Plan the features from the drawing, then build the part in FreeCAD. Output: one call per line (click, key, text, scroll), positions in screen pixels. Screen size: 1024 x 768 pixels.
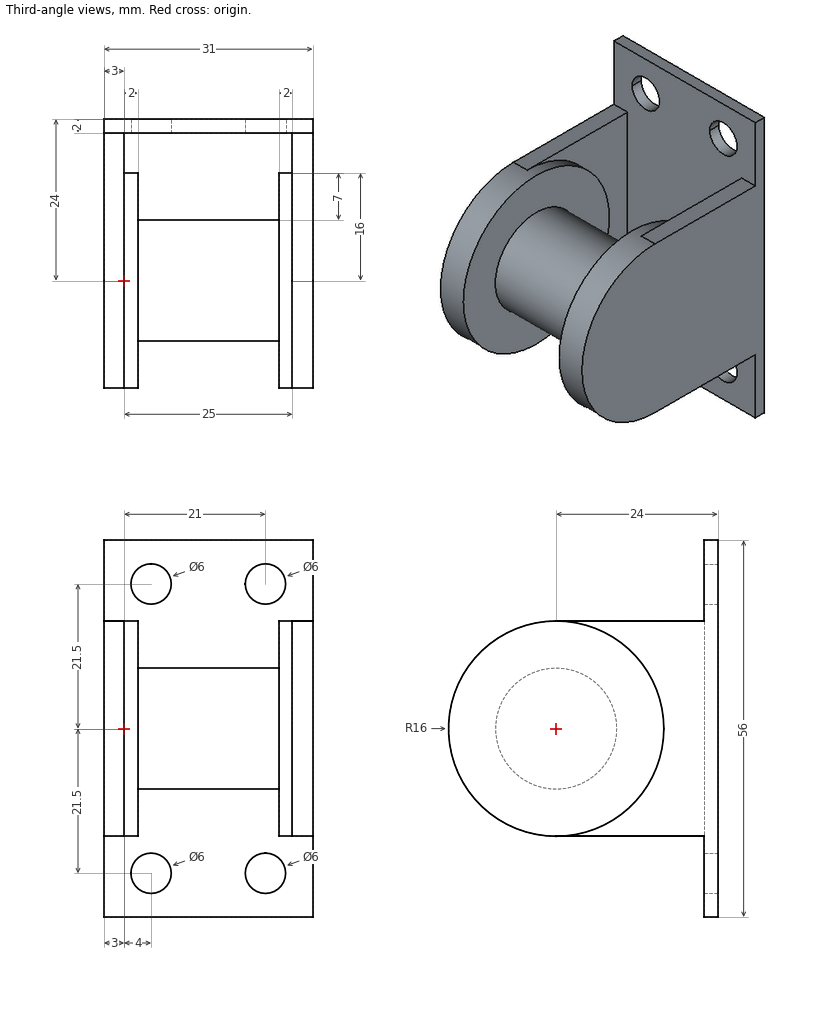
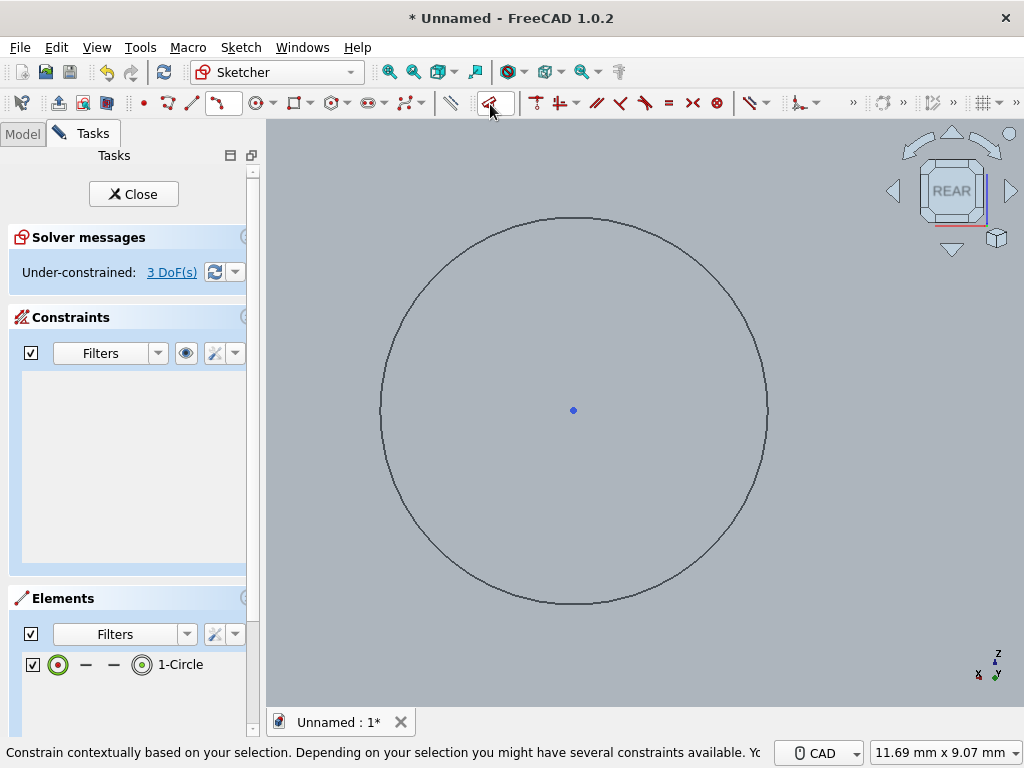
click(711, 274)
click(734, 251)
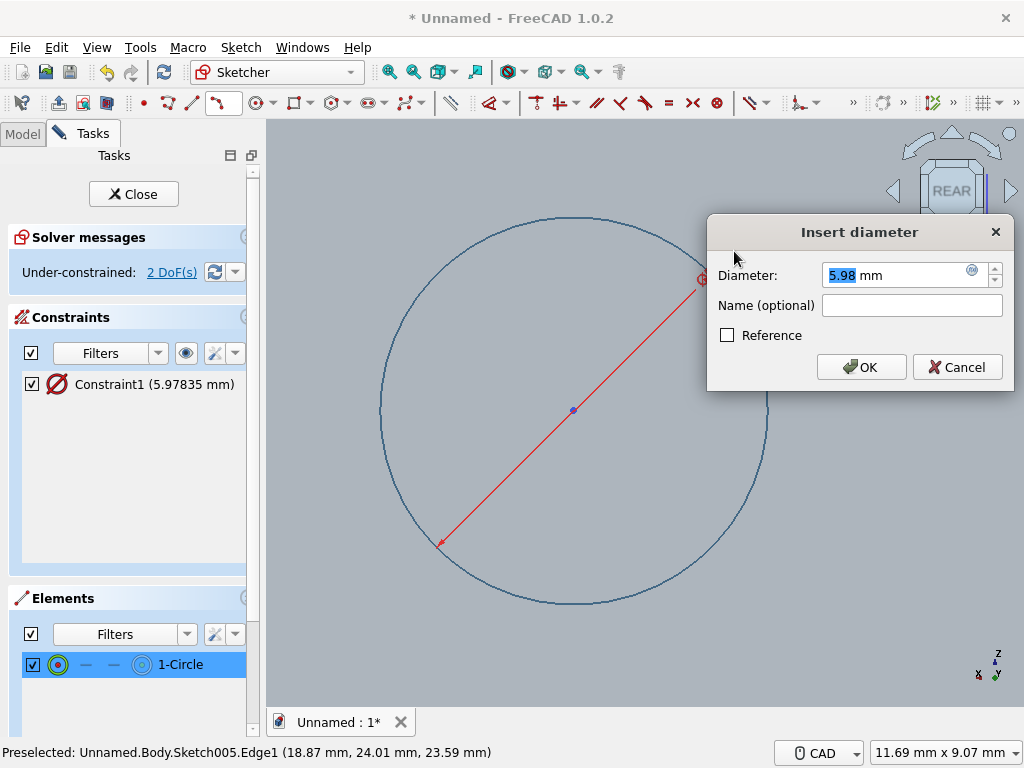
text(6)
key(Return)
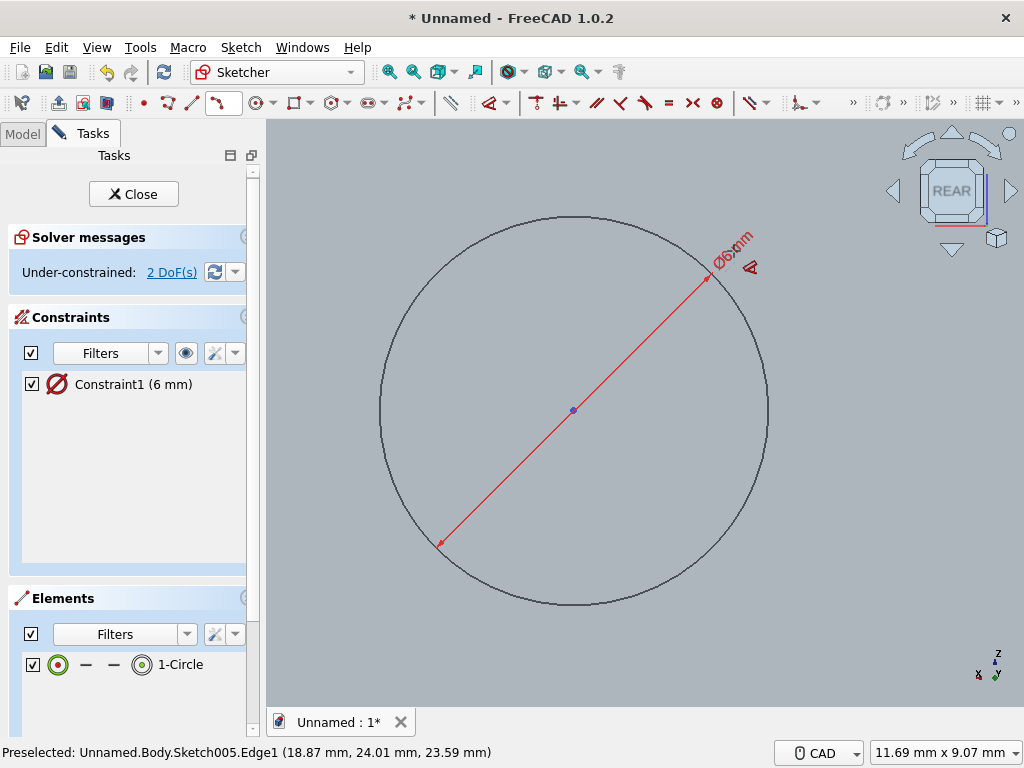
click(574, 411)
click(717, 377)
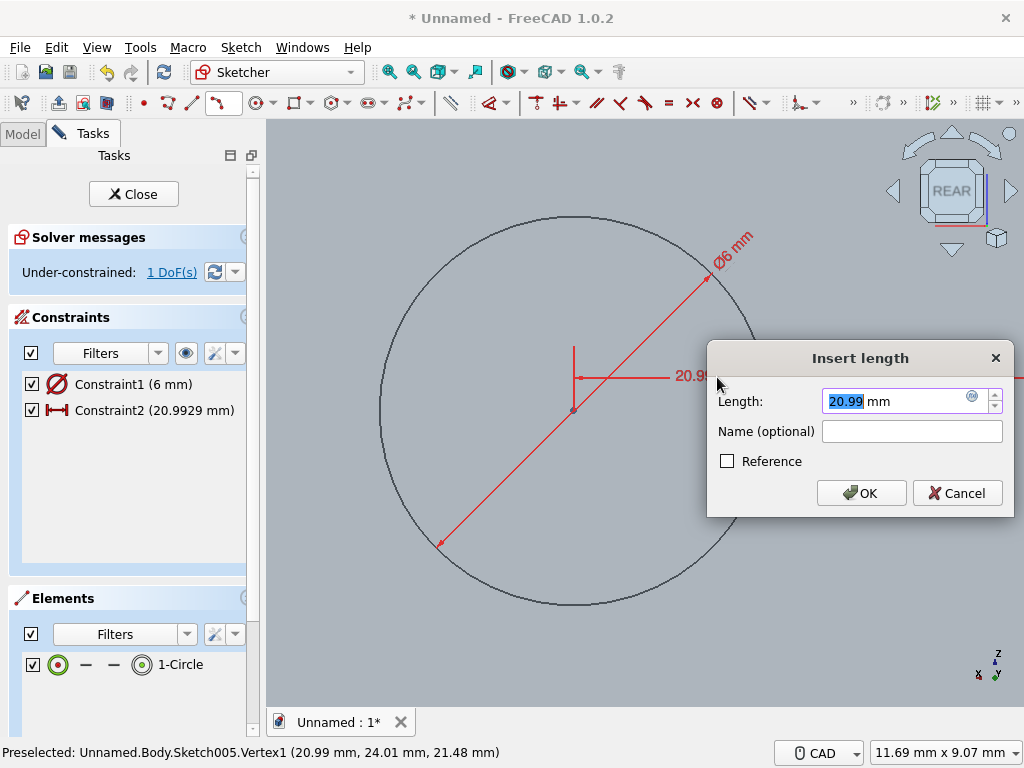
text(21)
key(Return)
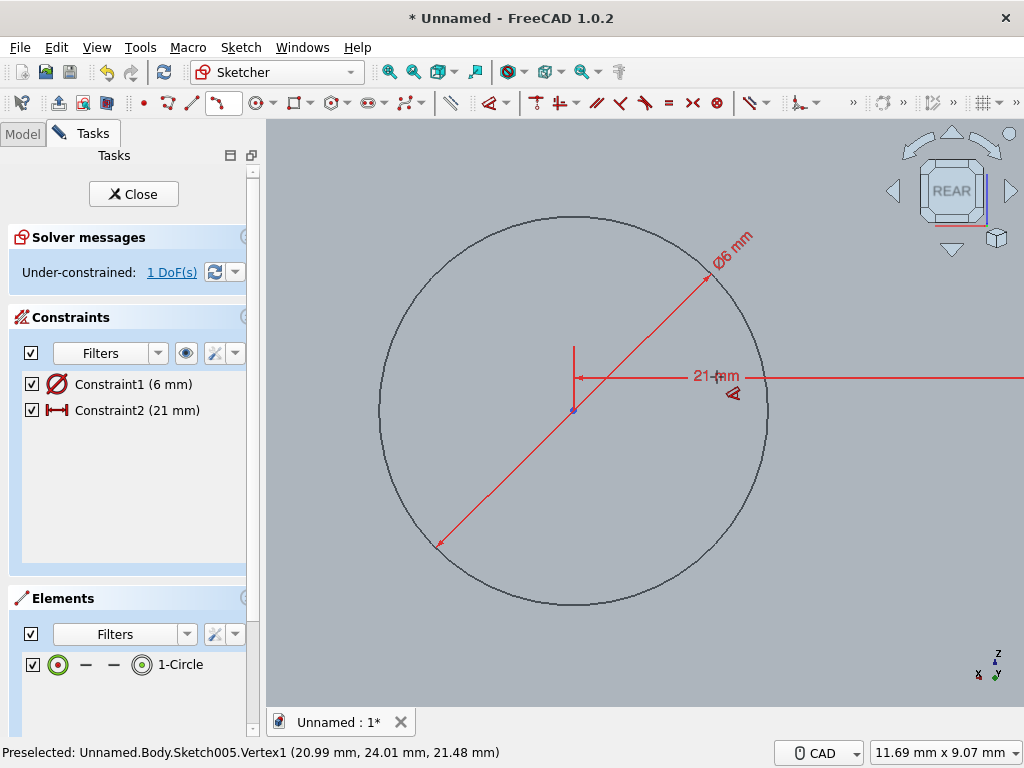
click(574, 411)
click(540, 545)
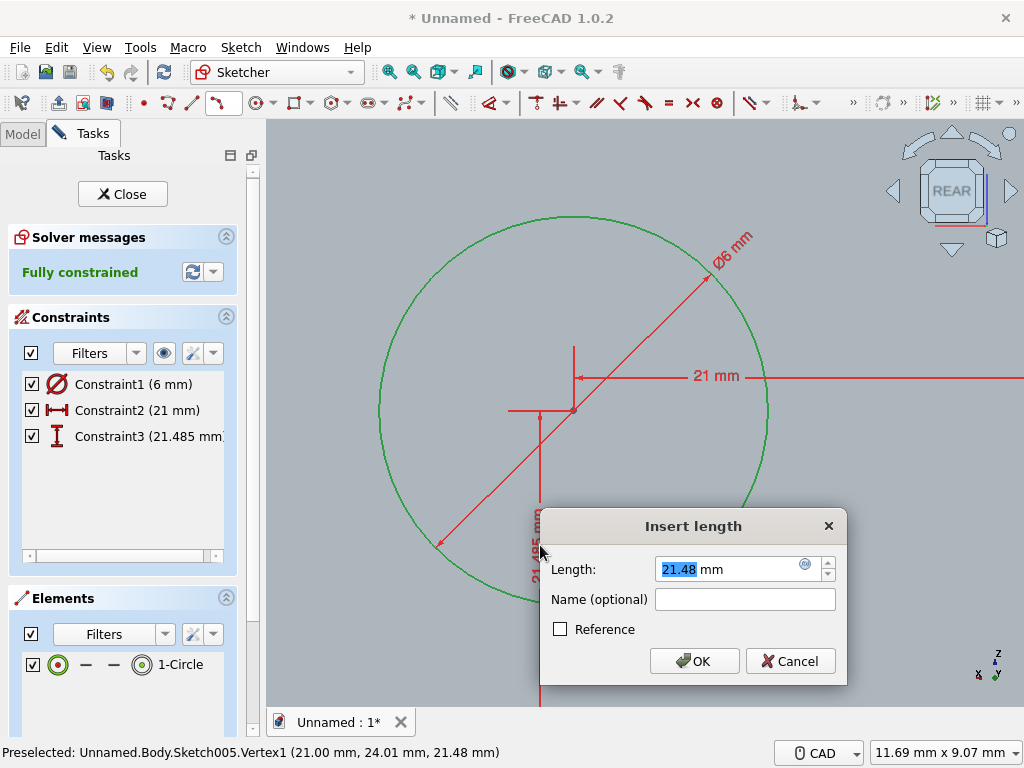
text(21.5)
key(Return)
key(Escape)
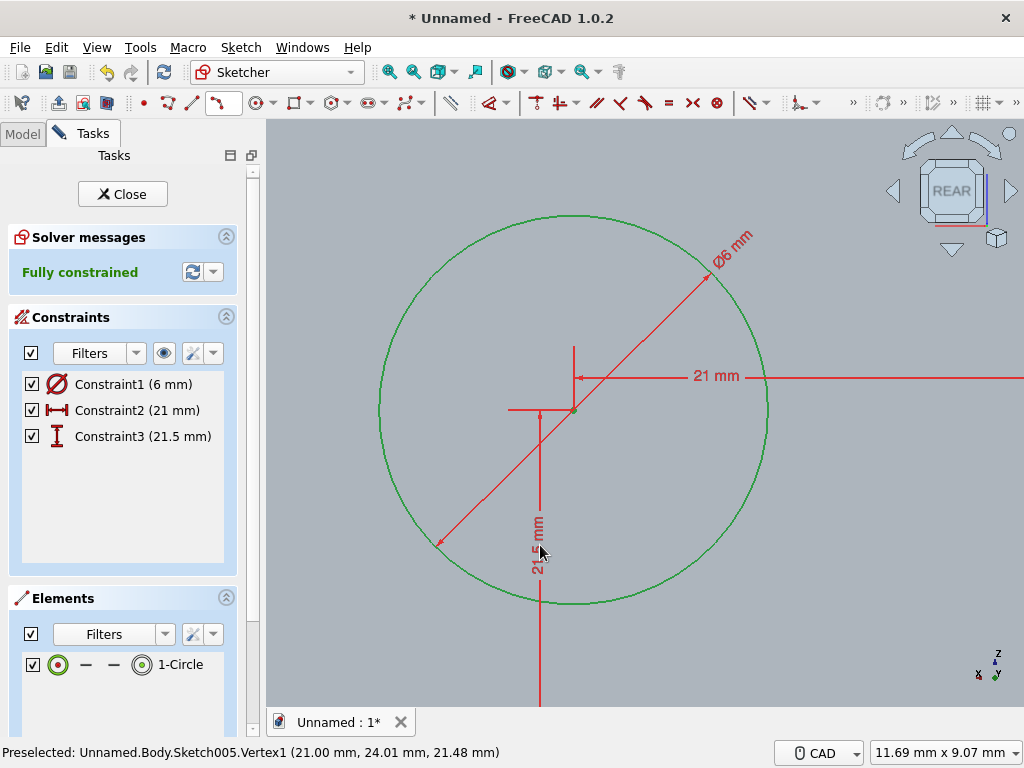
click(123, 194)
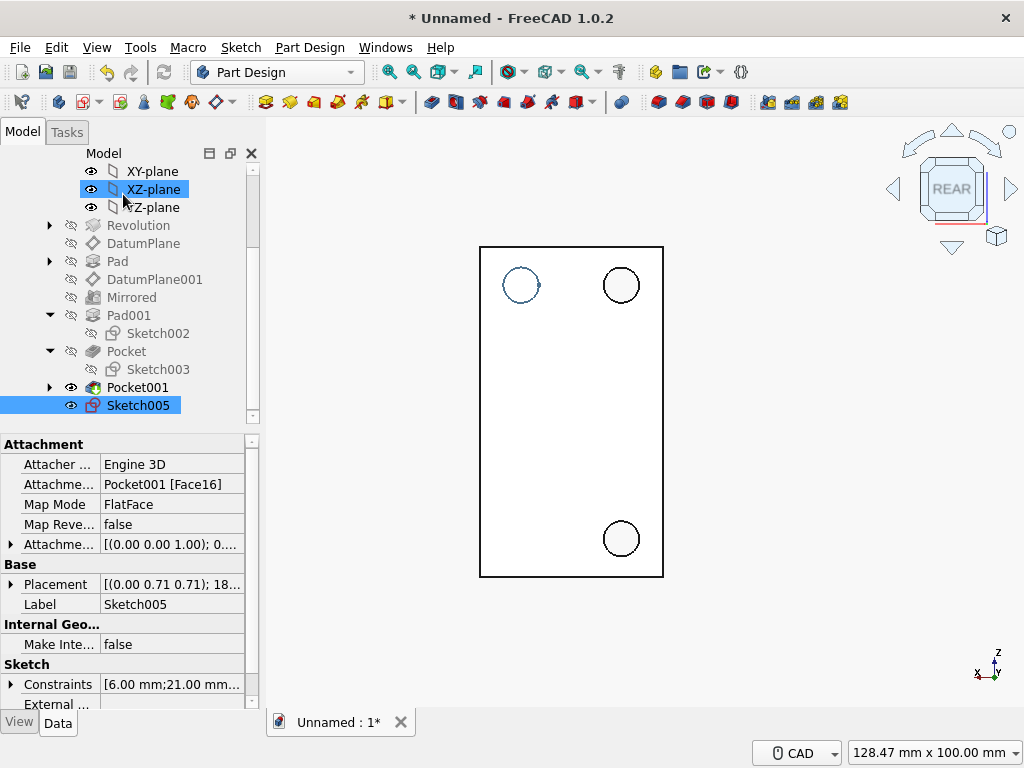
click(432, 102)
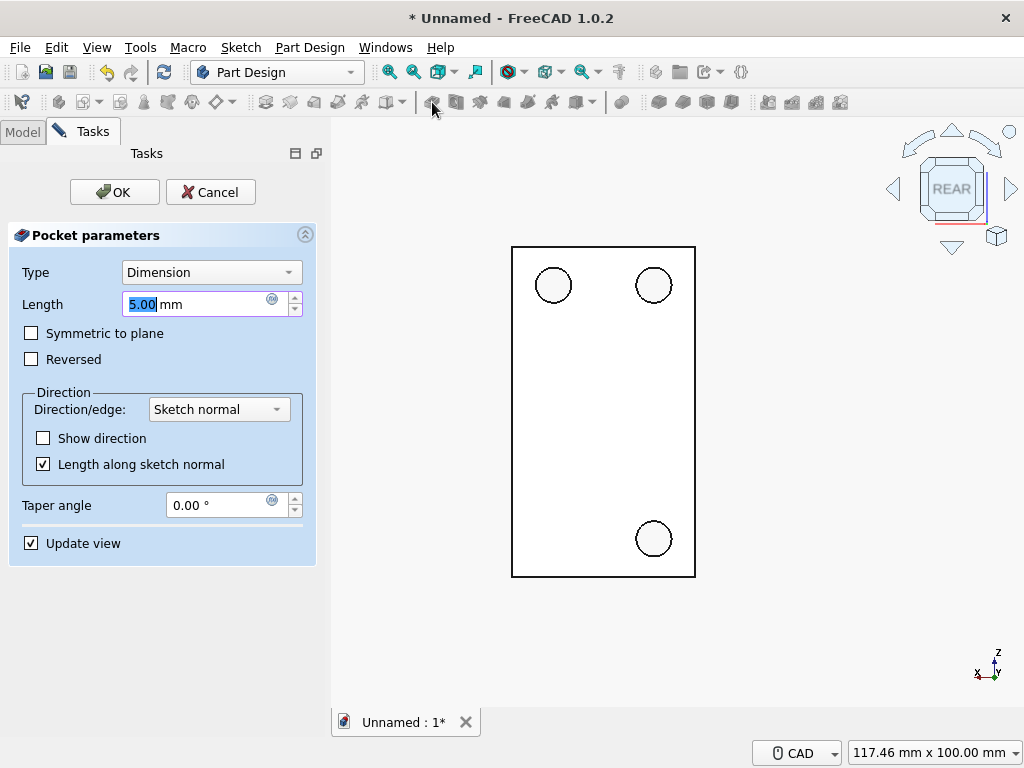
click(212, 272)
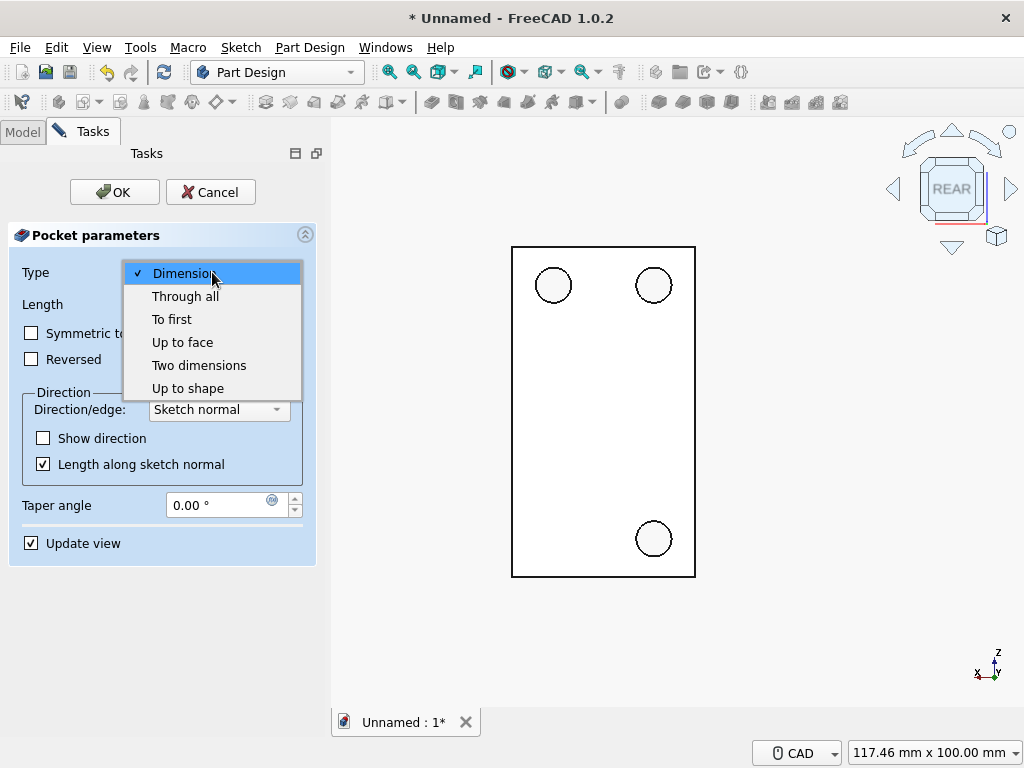
click(212, 320)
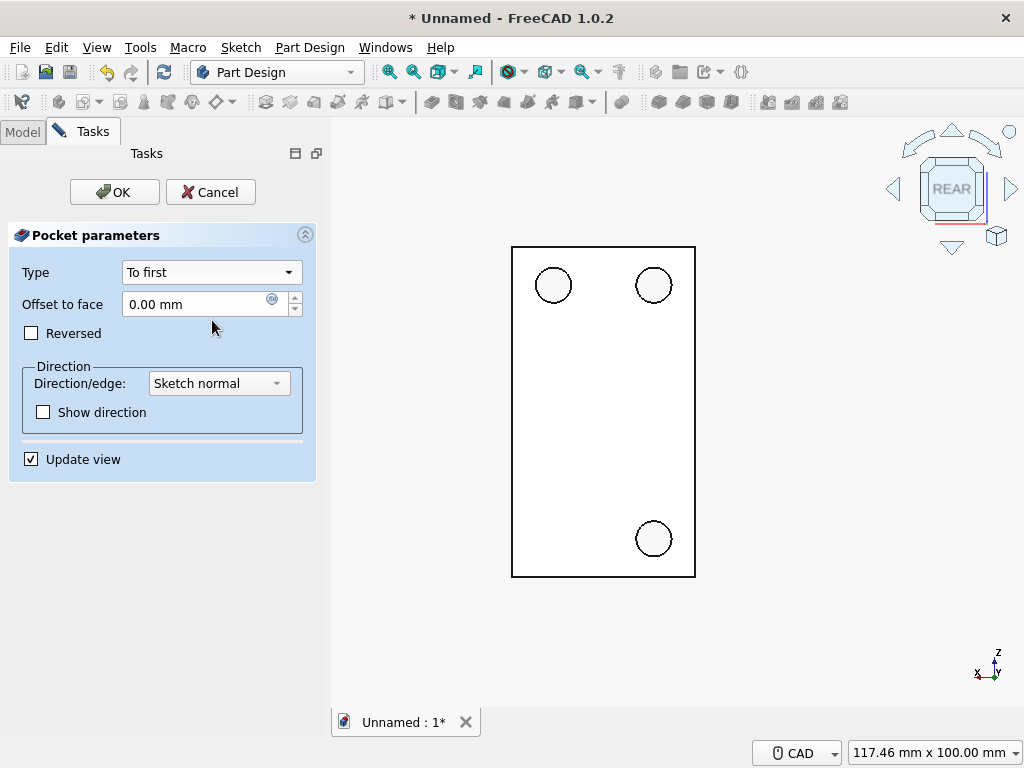
click(115, 192)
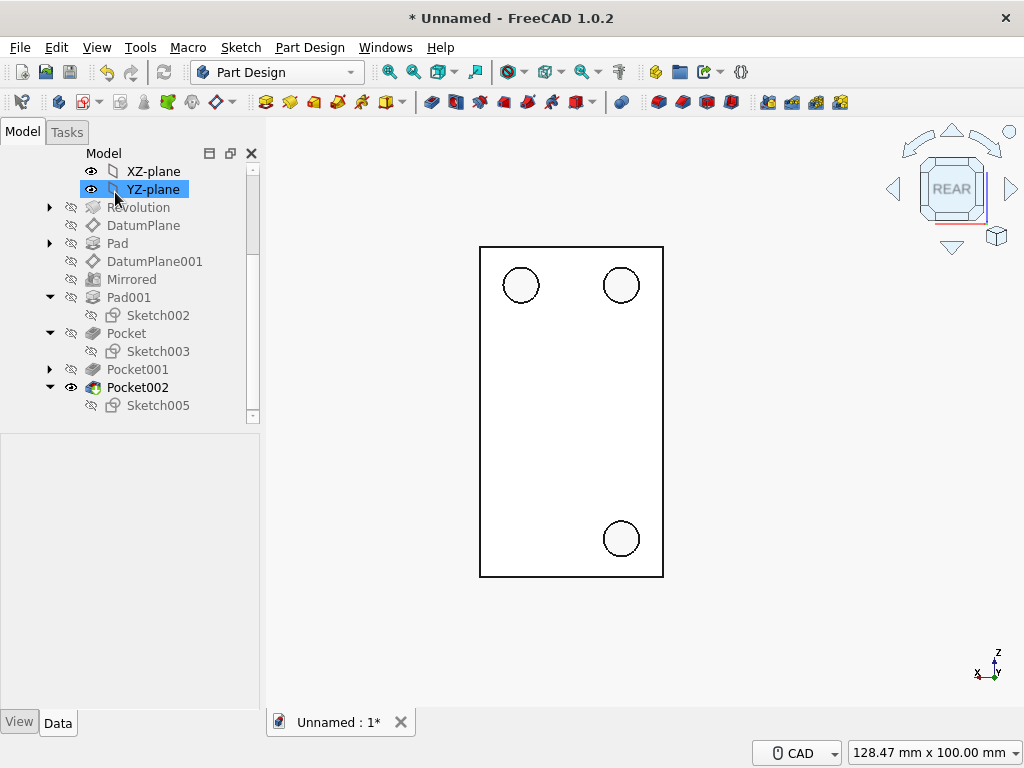
click(571, 411)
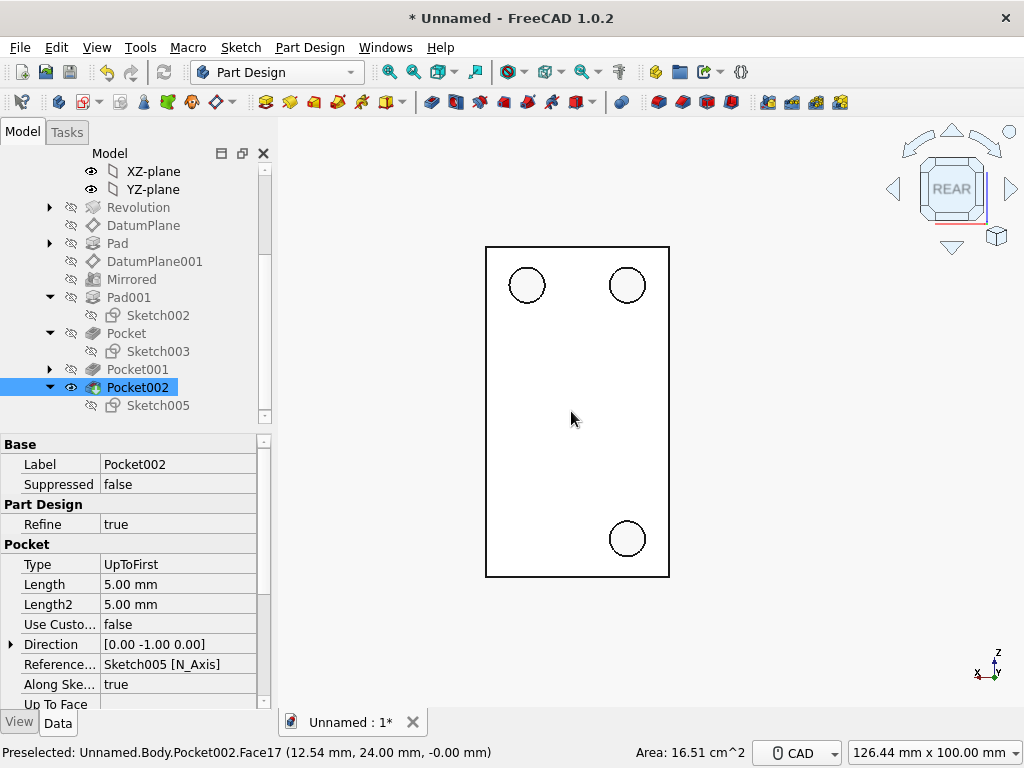
click(84, 102)